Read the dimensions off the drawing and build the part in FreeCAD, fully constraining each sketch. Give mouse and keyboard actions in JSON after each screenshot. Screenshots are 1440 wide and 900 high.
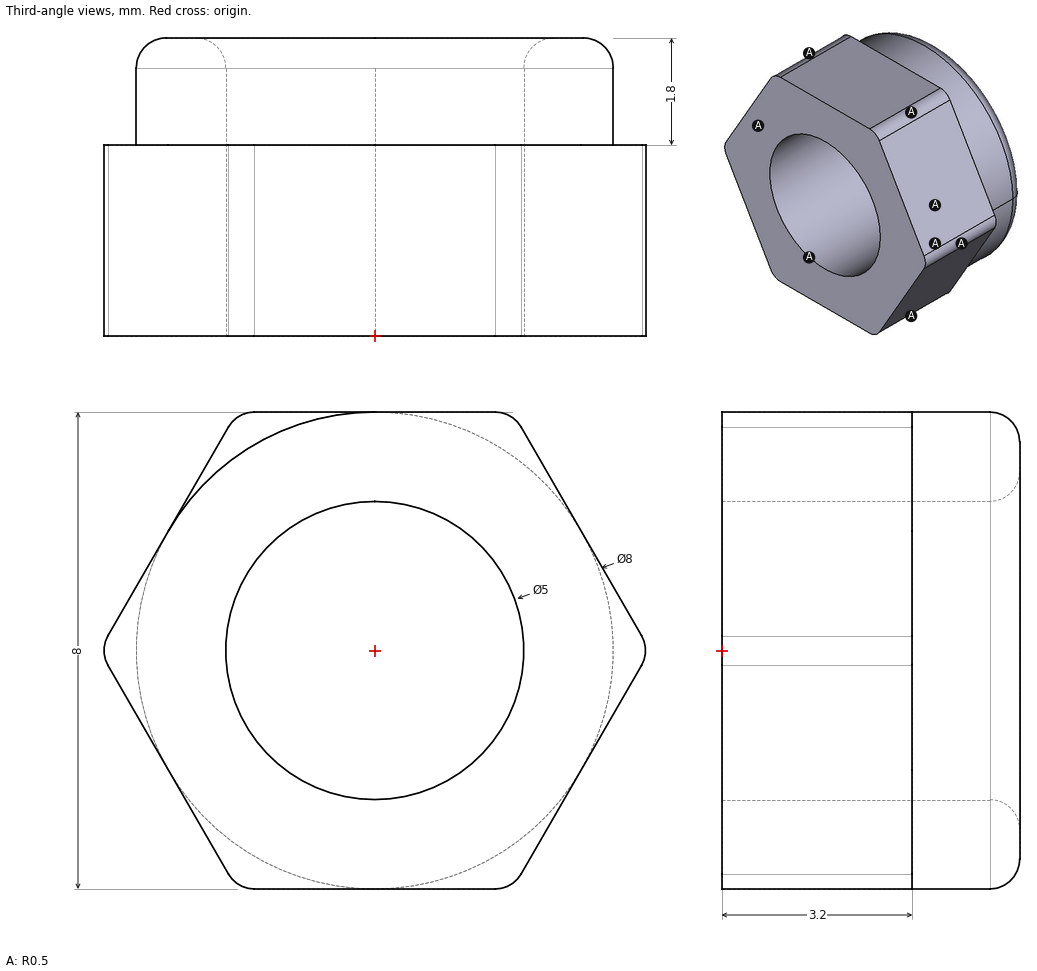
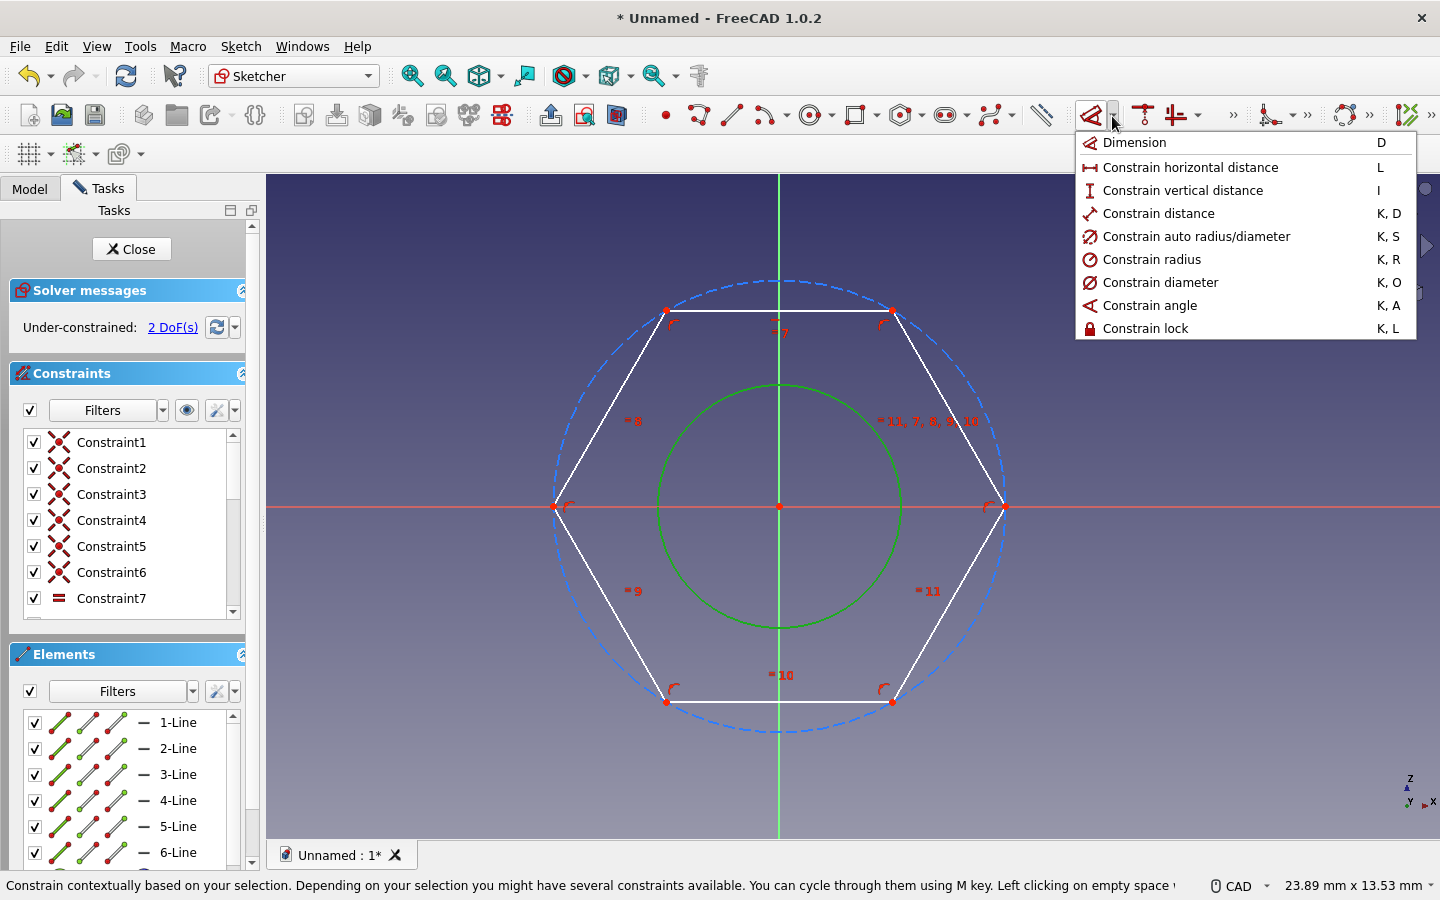
{"action": "left_click", "coordinate": [1246, 282]}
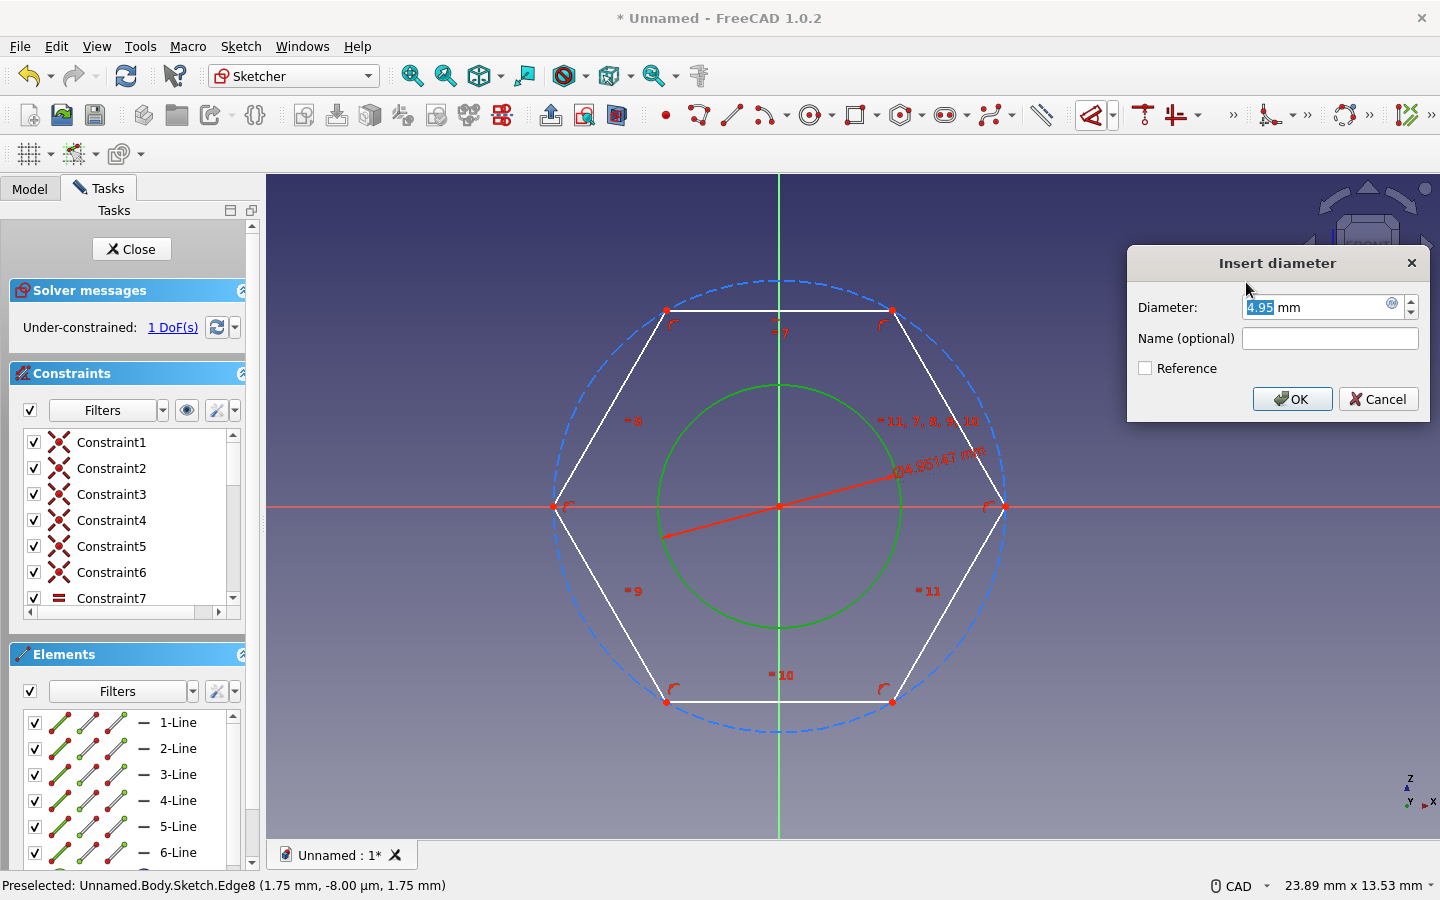
{"action": "type", "text": "5"}
{"action": "key", "text": "Return"}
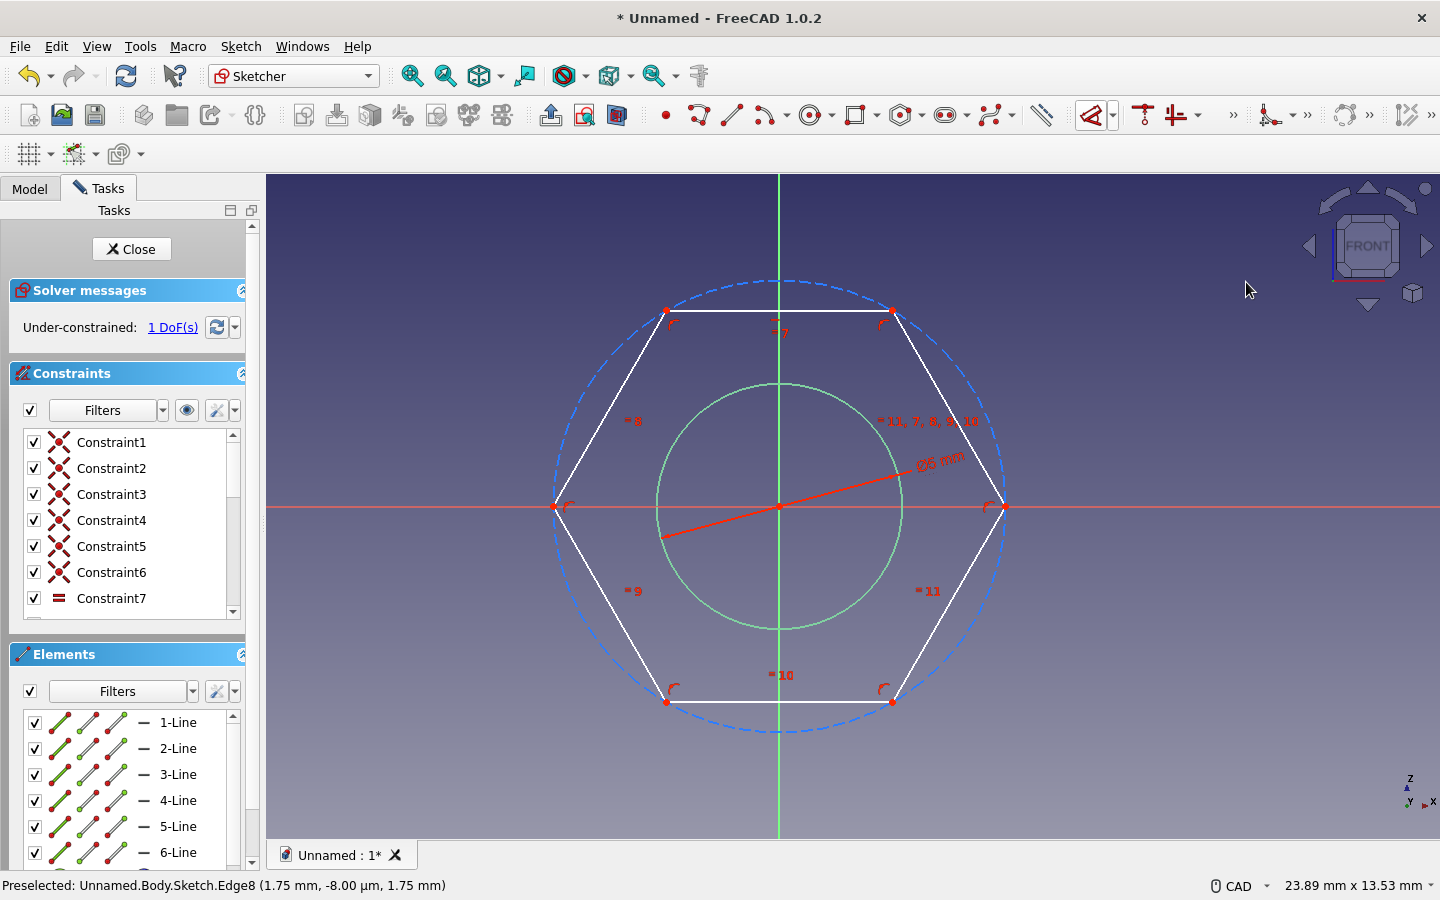
{"action": "left_click", "coordinate": [666, 702]}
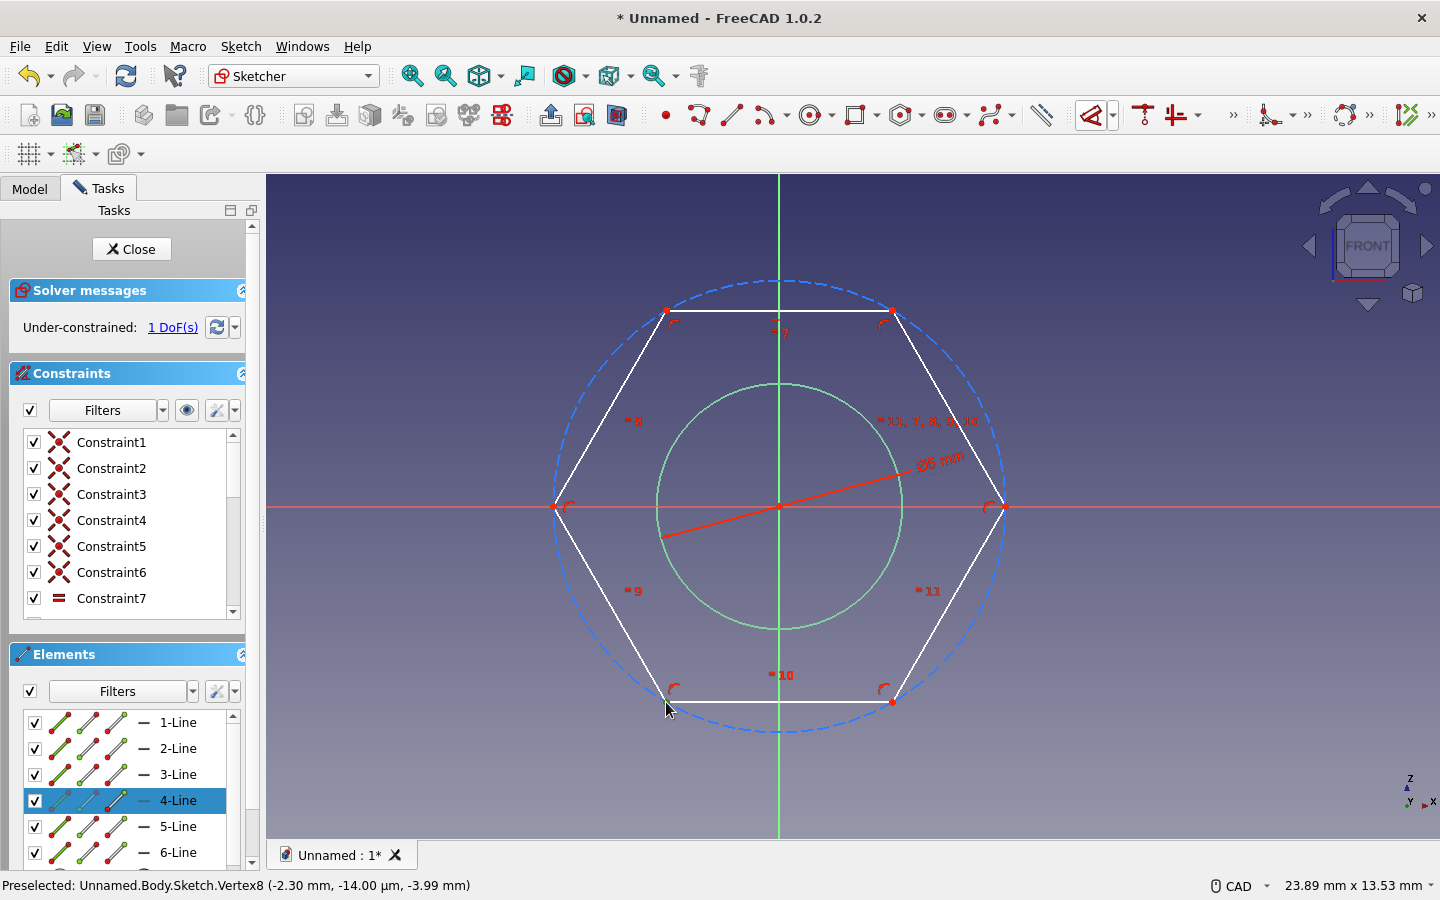
{"action": "left_click", "coordinate": [893, 311]}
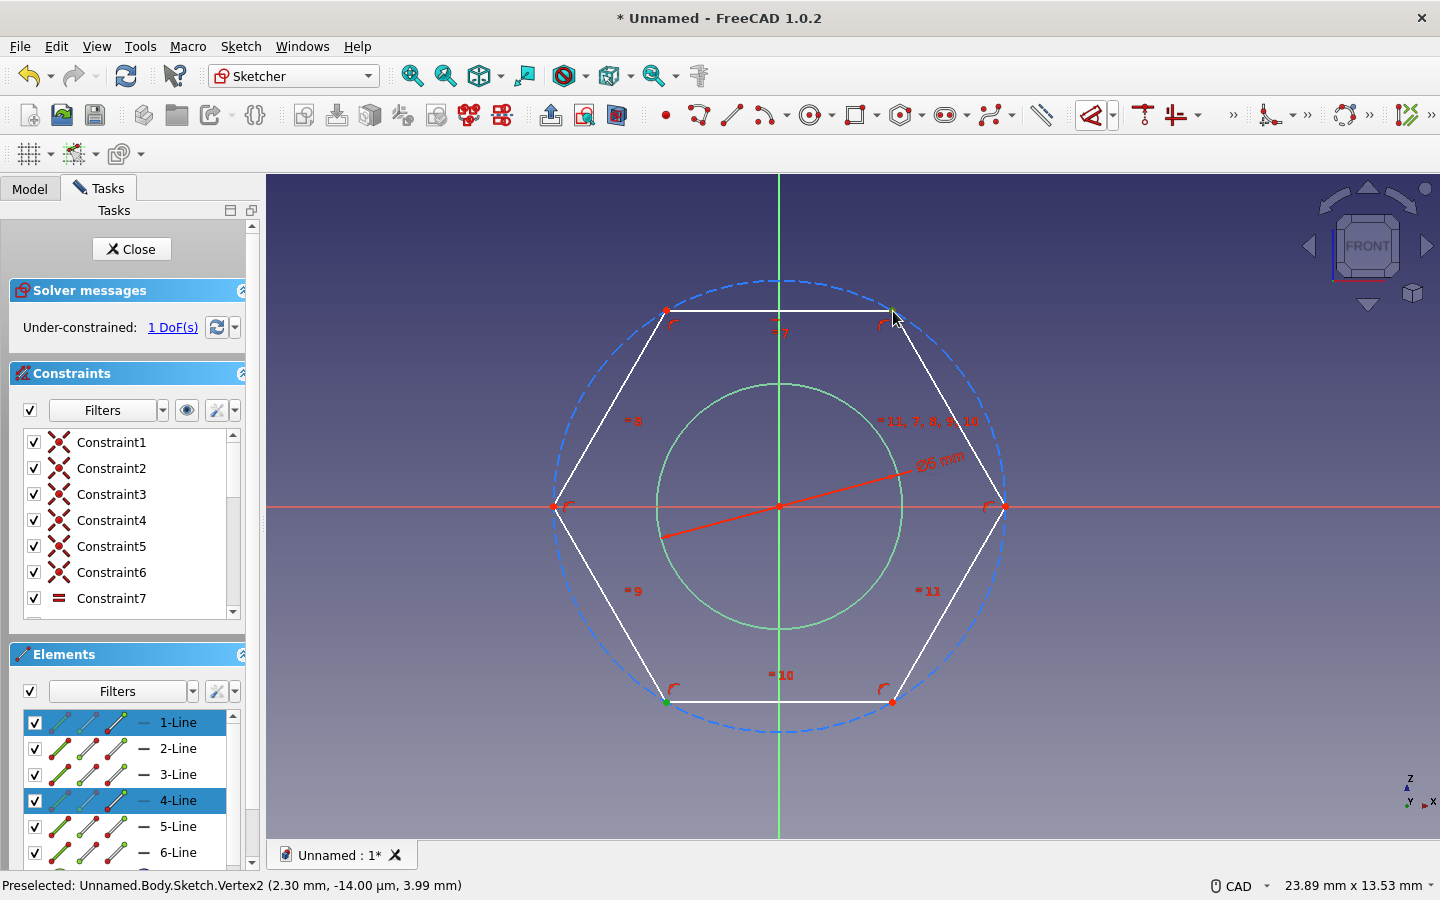
{"action": "left_click", "coordinate": [1112, 116]}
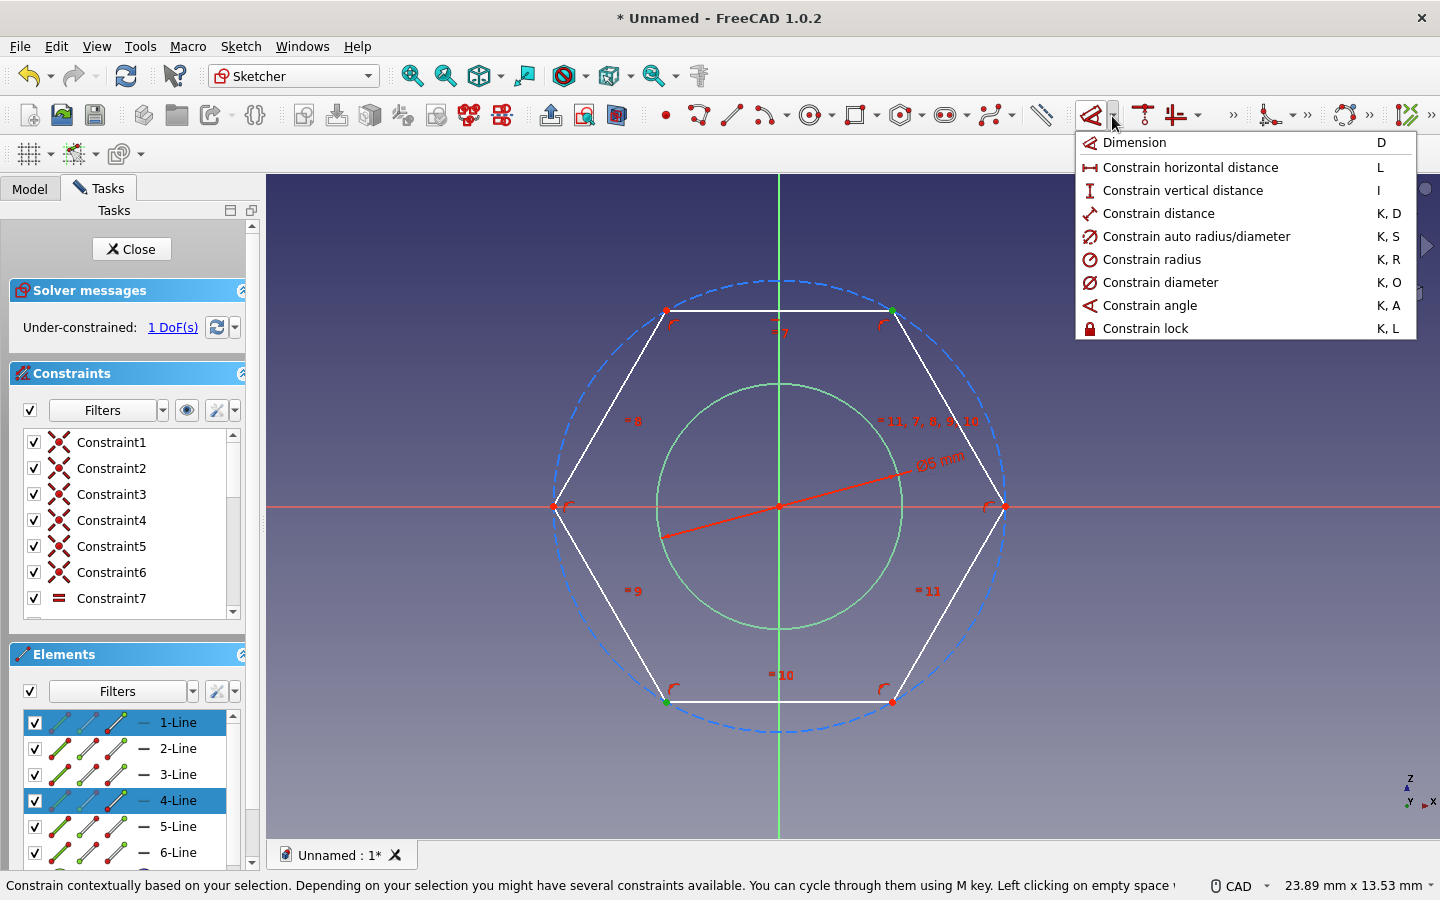
{"action": "left_click", "coordinate": [1246, 190]}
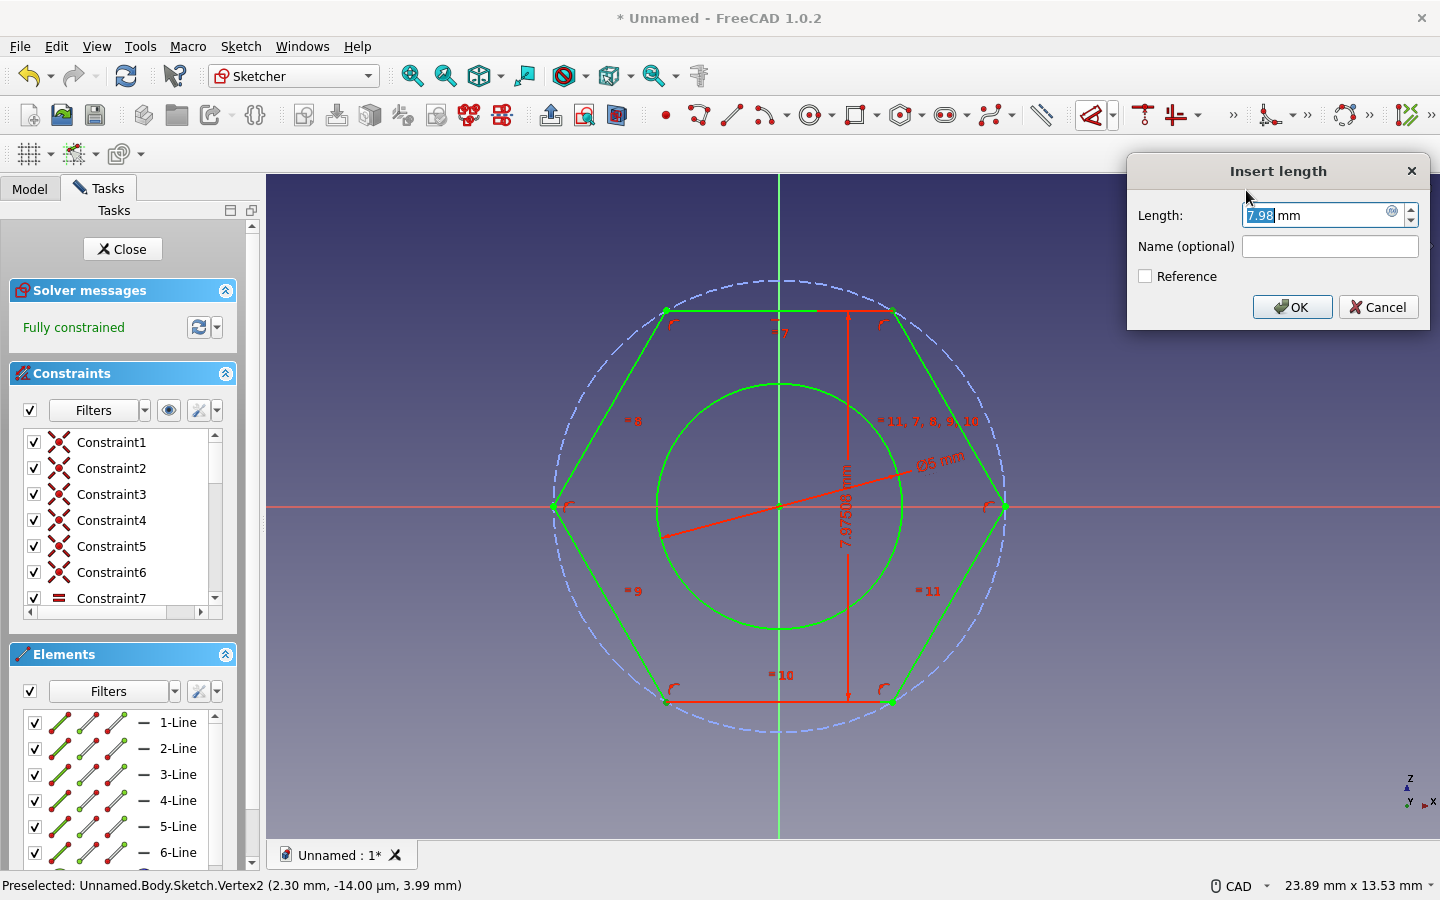
{"action": "type", "text": "8"}
{"action": "key", "text": "Return"}